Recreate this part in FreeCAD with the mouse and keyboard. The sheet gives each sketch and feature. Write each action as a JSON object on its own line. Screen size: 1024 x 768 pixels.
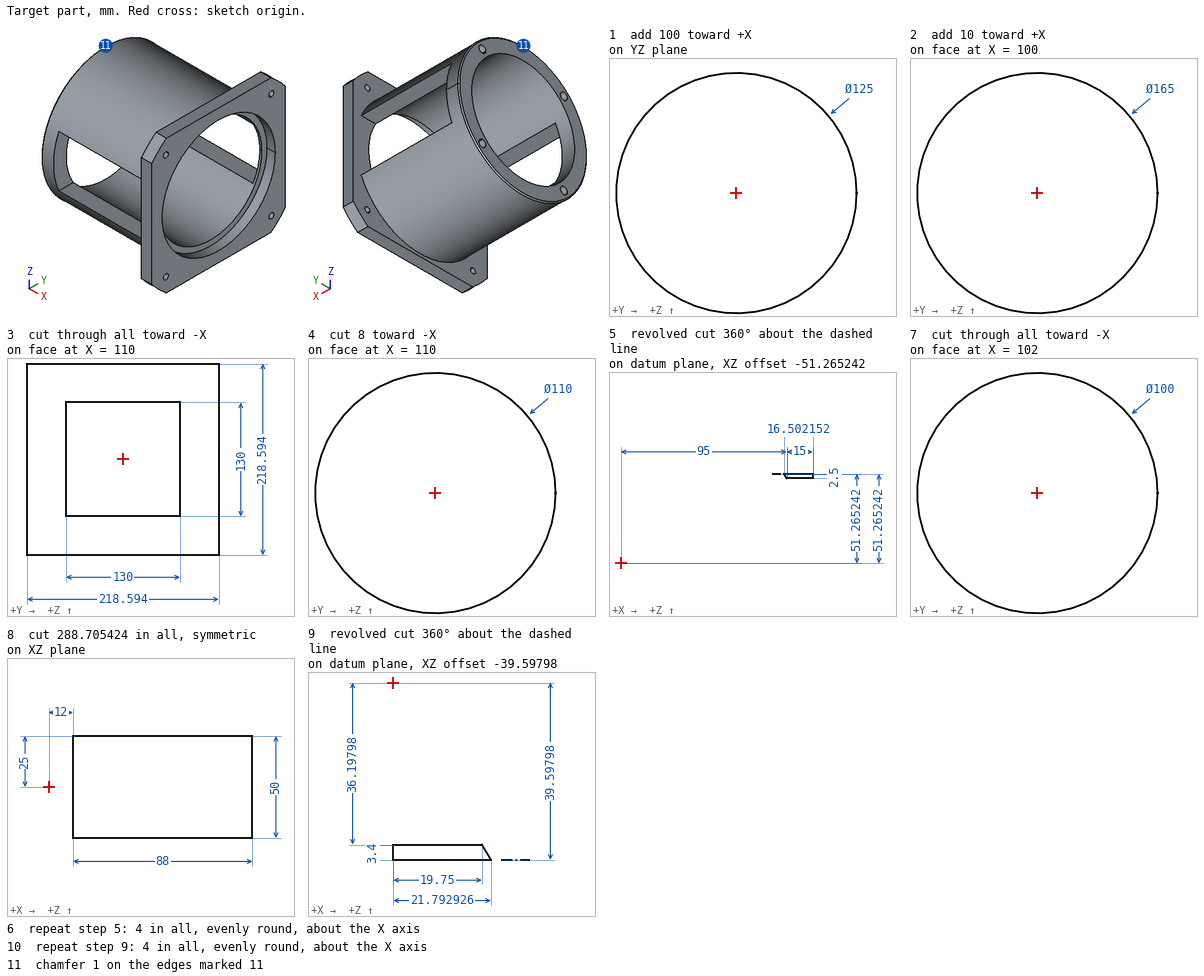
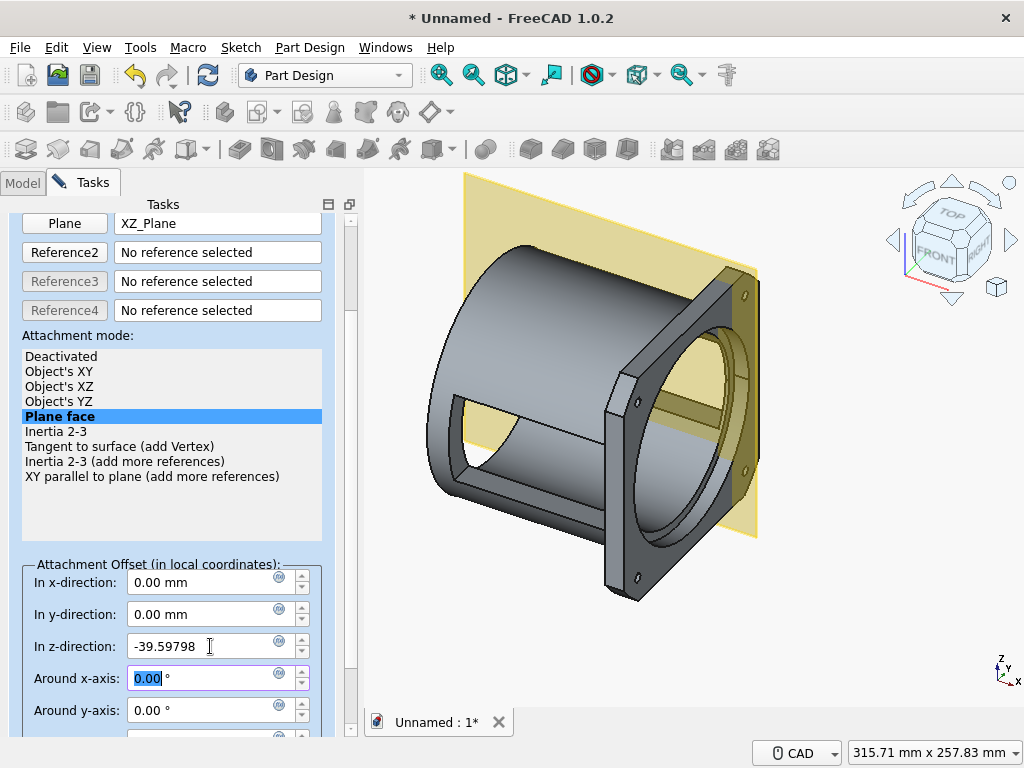
{"action": "scroll", "coordinate": [351, 475], "scroll_direction": "up", "scroll_amount": 3}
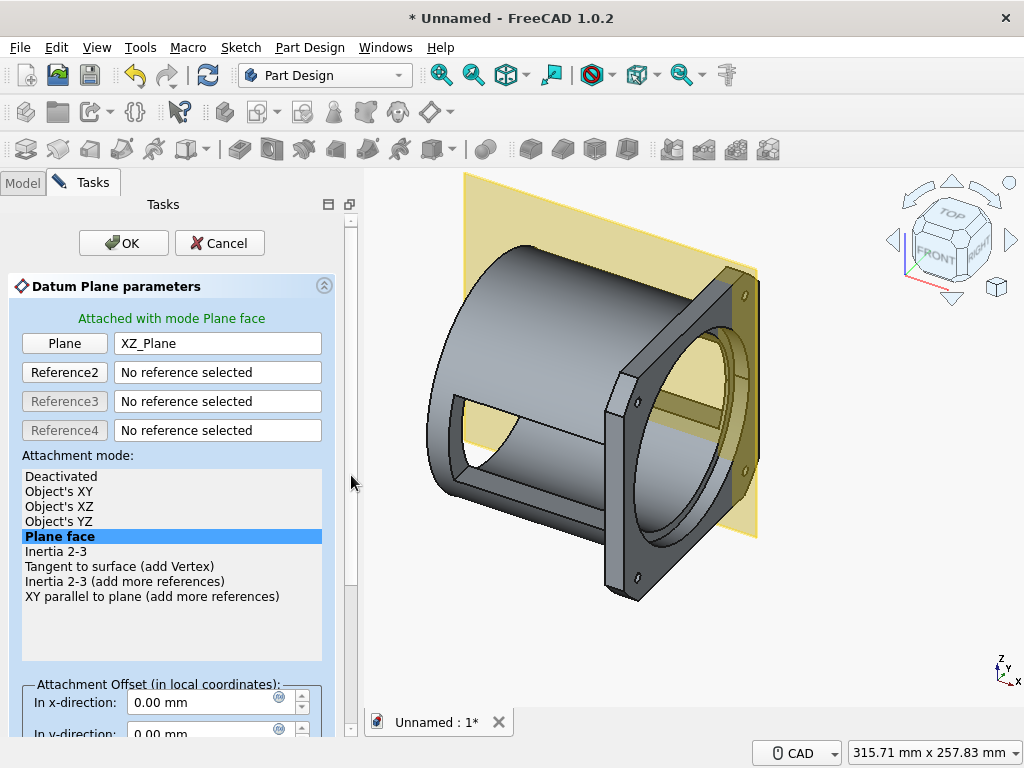
{"action": "left_click", "coordinate": [124, 243]}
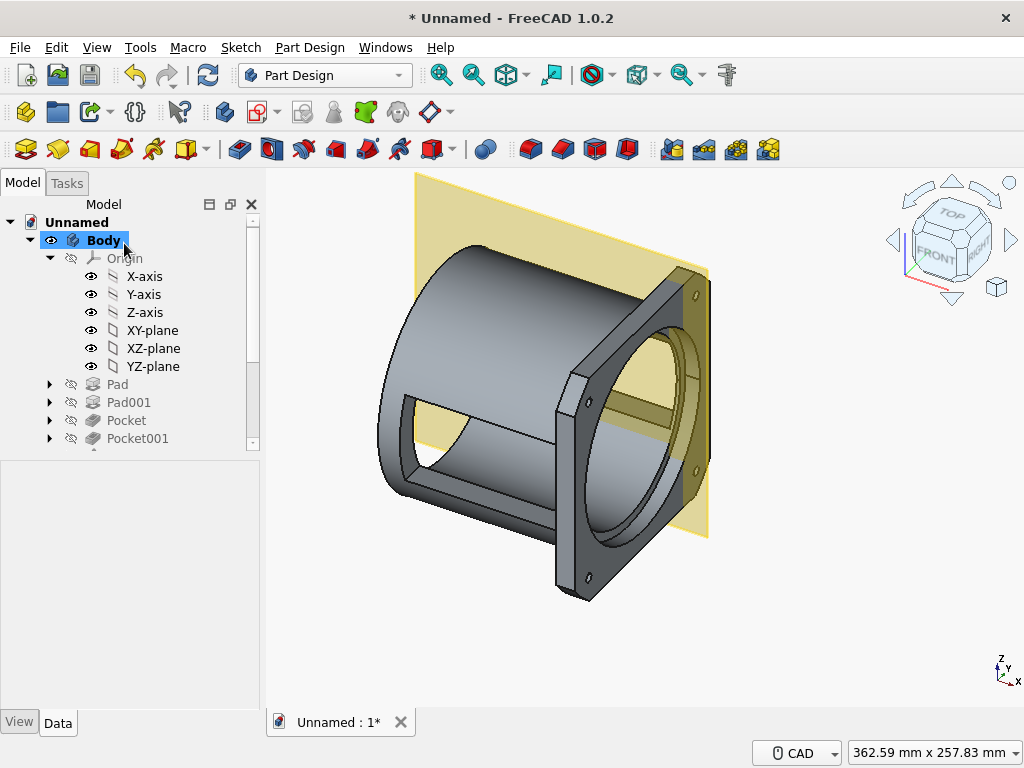
{"action": "scroll", "coordinate": [100, 326], "scroll_direction": "down", "scroll_amount": 3}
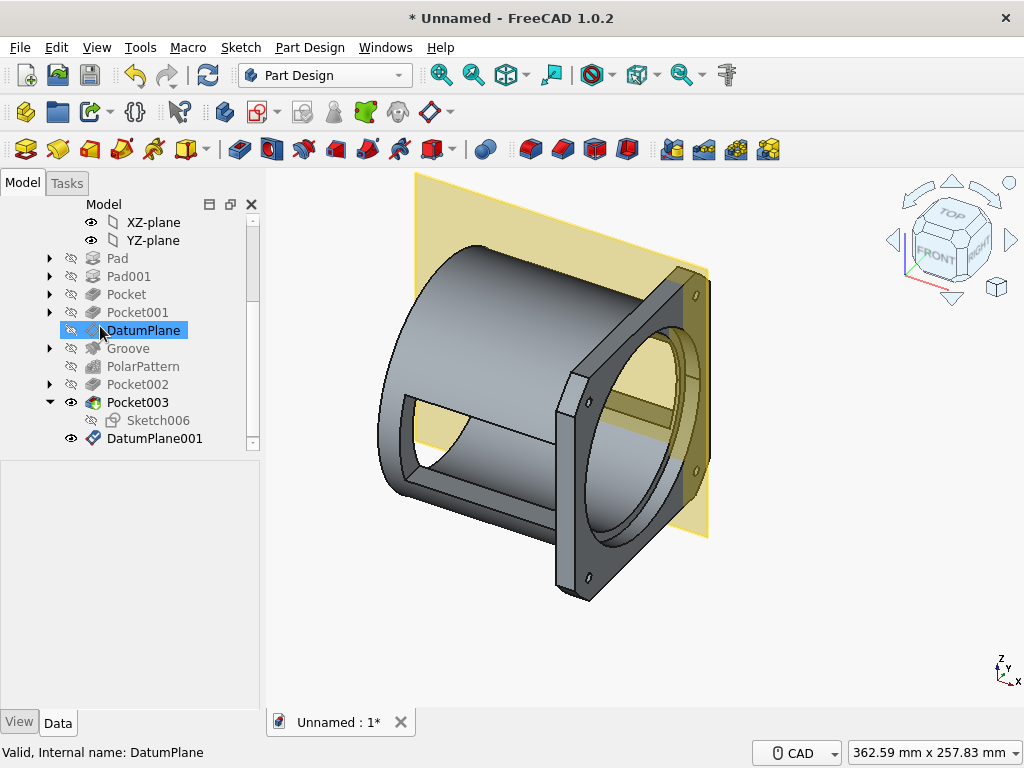
{"action": "left_click", "coordinate": [116, 438]}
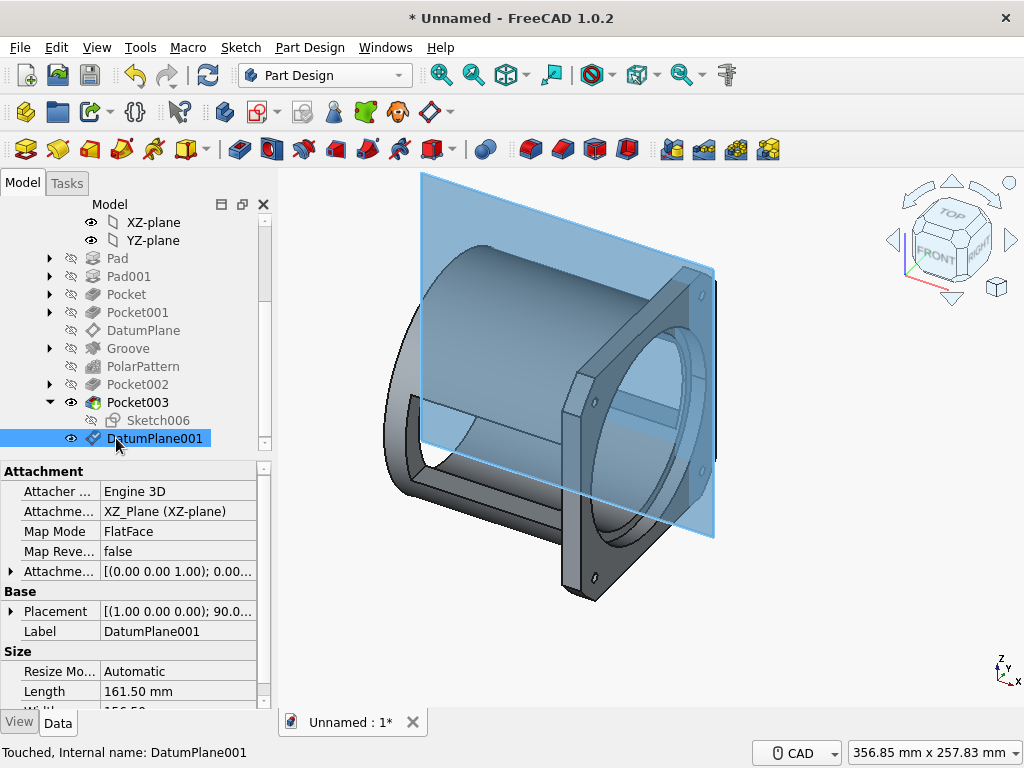
{"action": "left_click", "coordinate": [258, 112]}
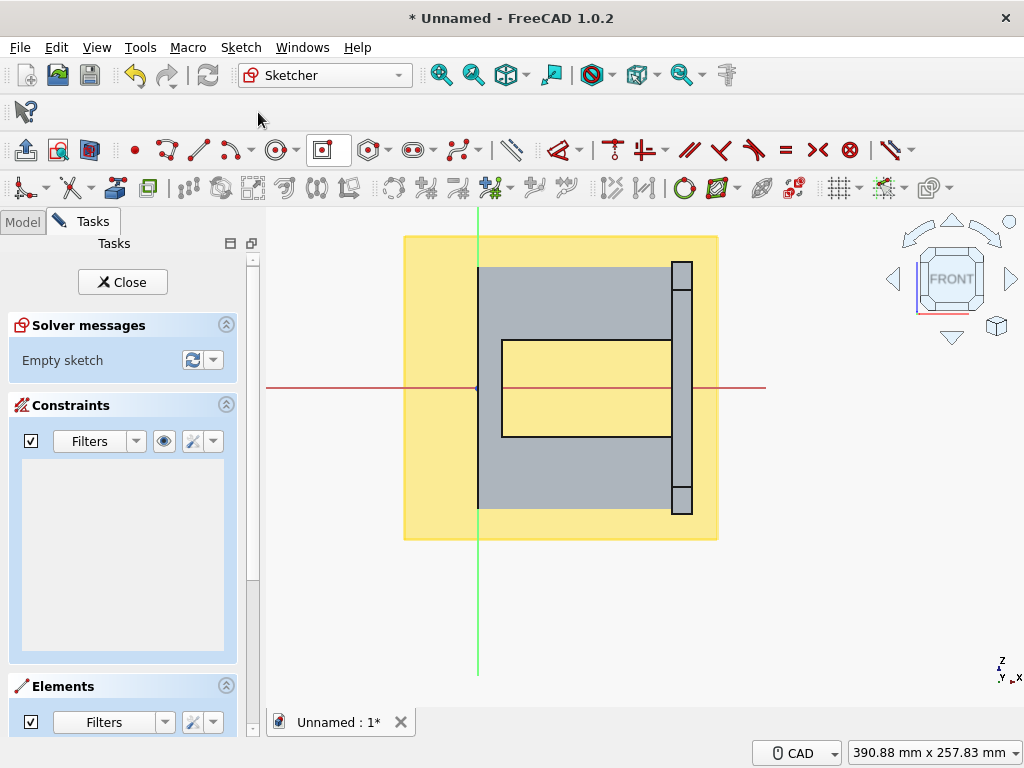
{"action": "left_click", "coordinate": [90, 150]}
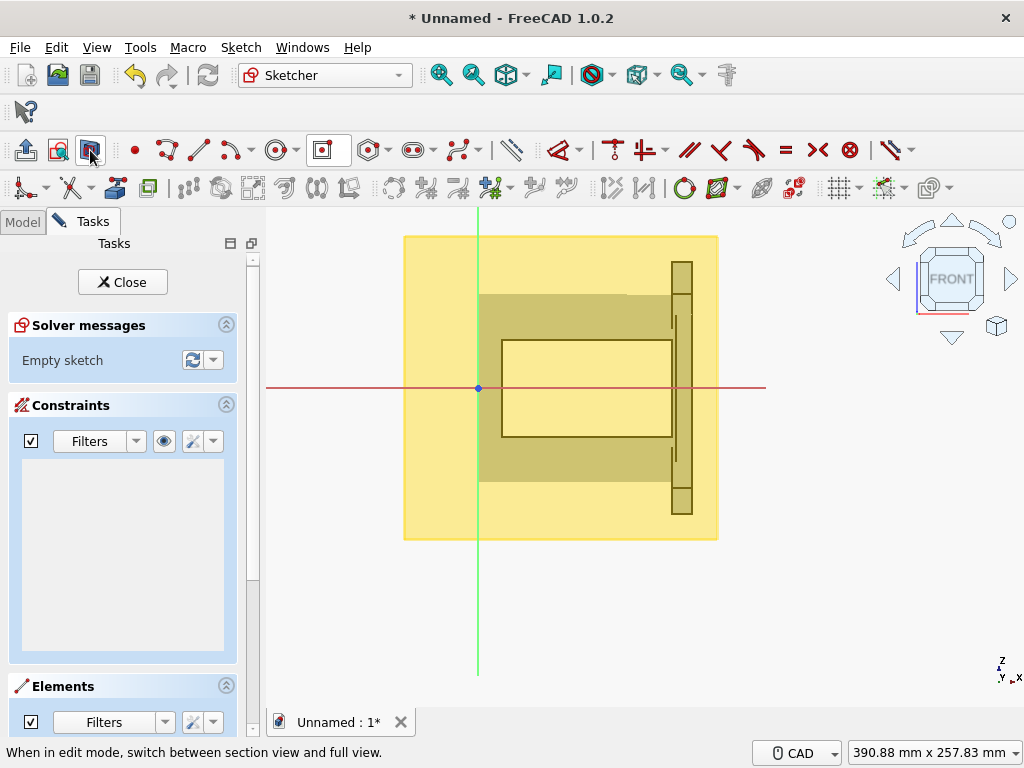
{"action": "scroll", "coordinate": [485, 417], "scroll_direction": "up", "scroll_amount": 7}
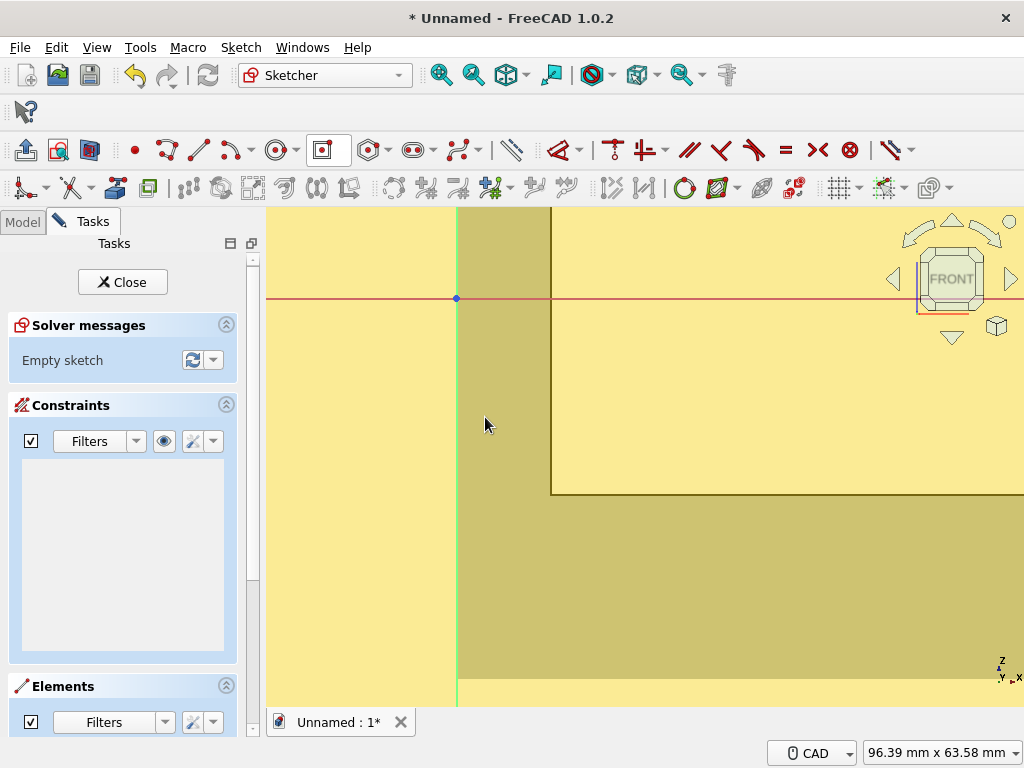
{"action": "left_click", "coordinate": [168, 150]}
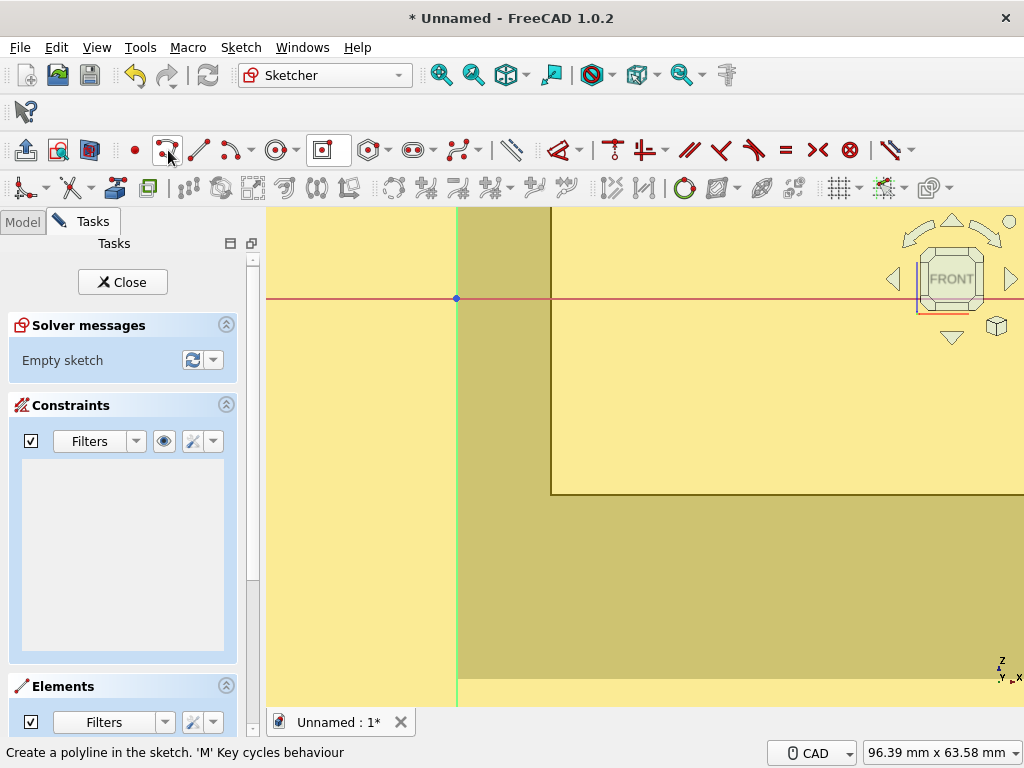
{"action": "left_click", "coordinate": [457, 584]}
{"action": "left_click", "coordinate": [612, 584]}
{"action": "left_click", "coordinate": [628, 610]}
{"action": "left_click", "coordinate": [466, 610]}
{"action": "left_click", "coordinate": [457, 585]}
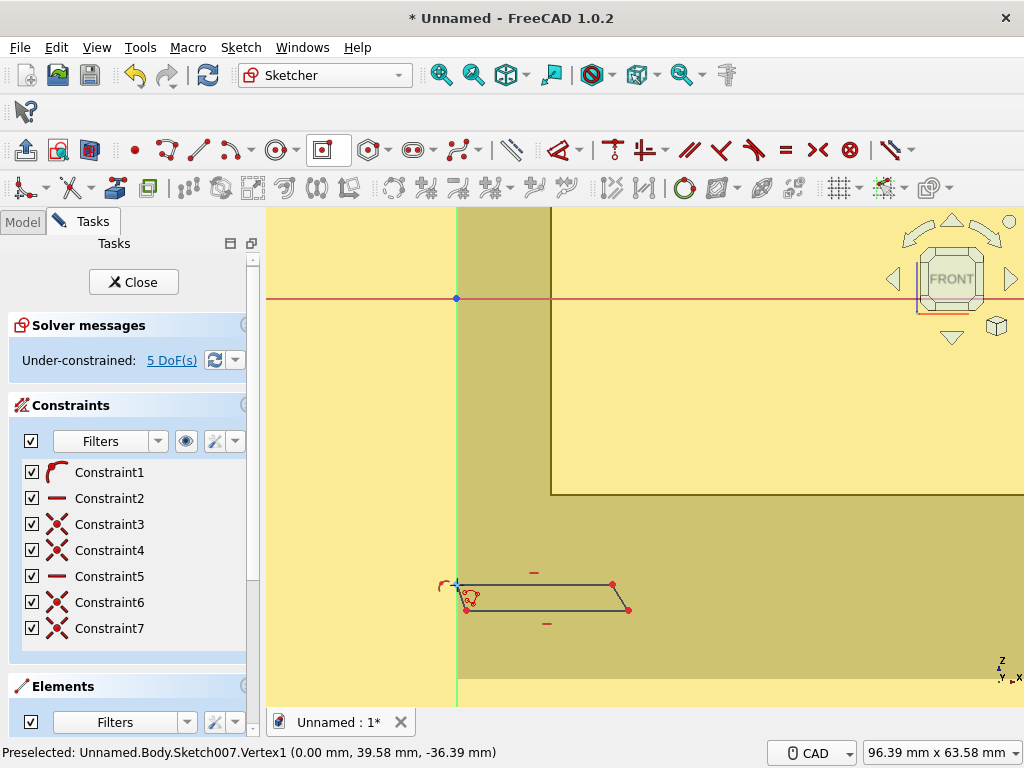
{"action": "left_click", "coordinate": [200, 150]}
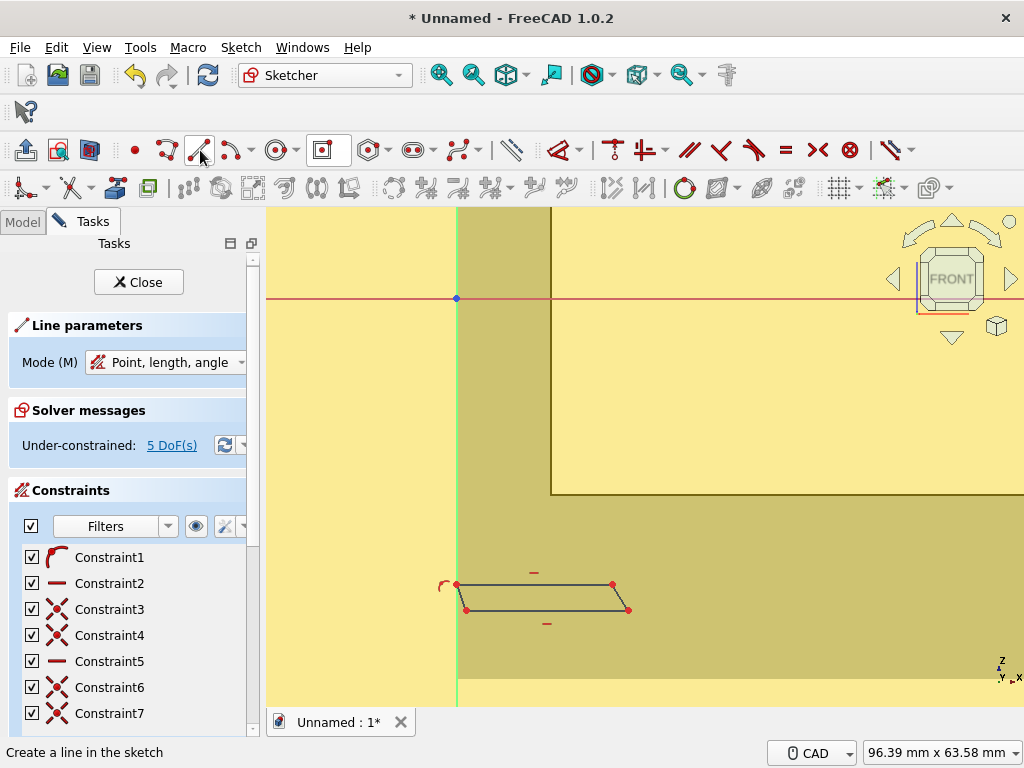
{"action": "left_click", "coordinate": [645, 610]}
{"action": "left_click", "coordinate": [697, 610]}
{"action": "key", "text": "Escape"}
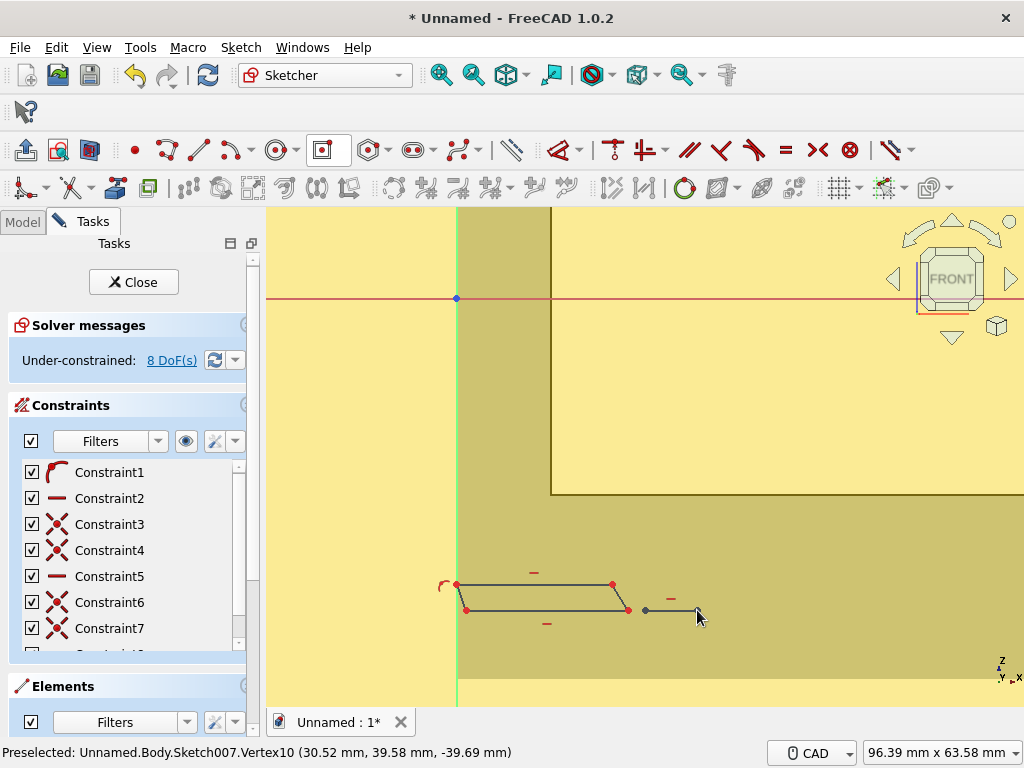
{"action": "left_click", "coordinate": [661, 611]}